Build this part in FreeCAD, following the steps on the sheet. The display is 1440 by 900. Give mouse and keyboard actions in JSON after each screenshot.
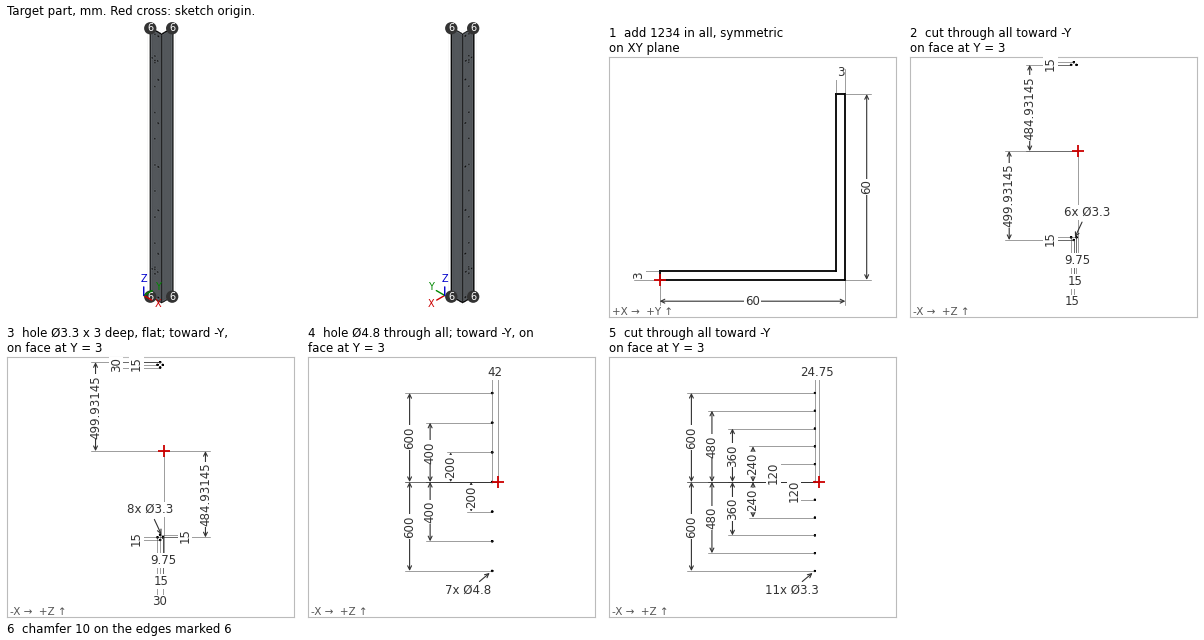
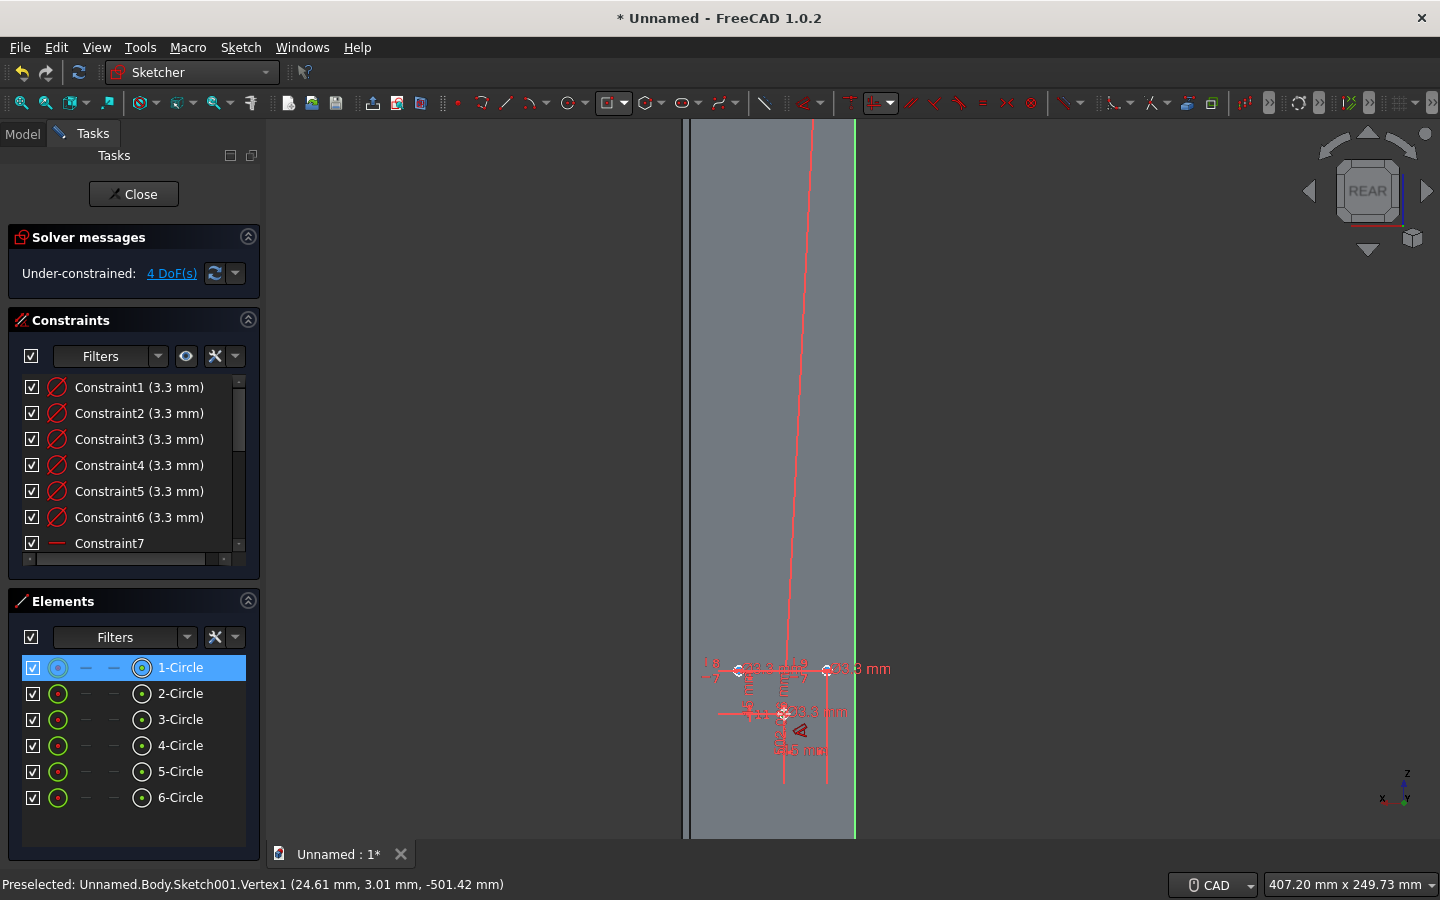
{"action": "left_click", "coordinate": [739, 671]}
{"action": "left_click", "coordinate": [761, 637]}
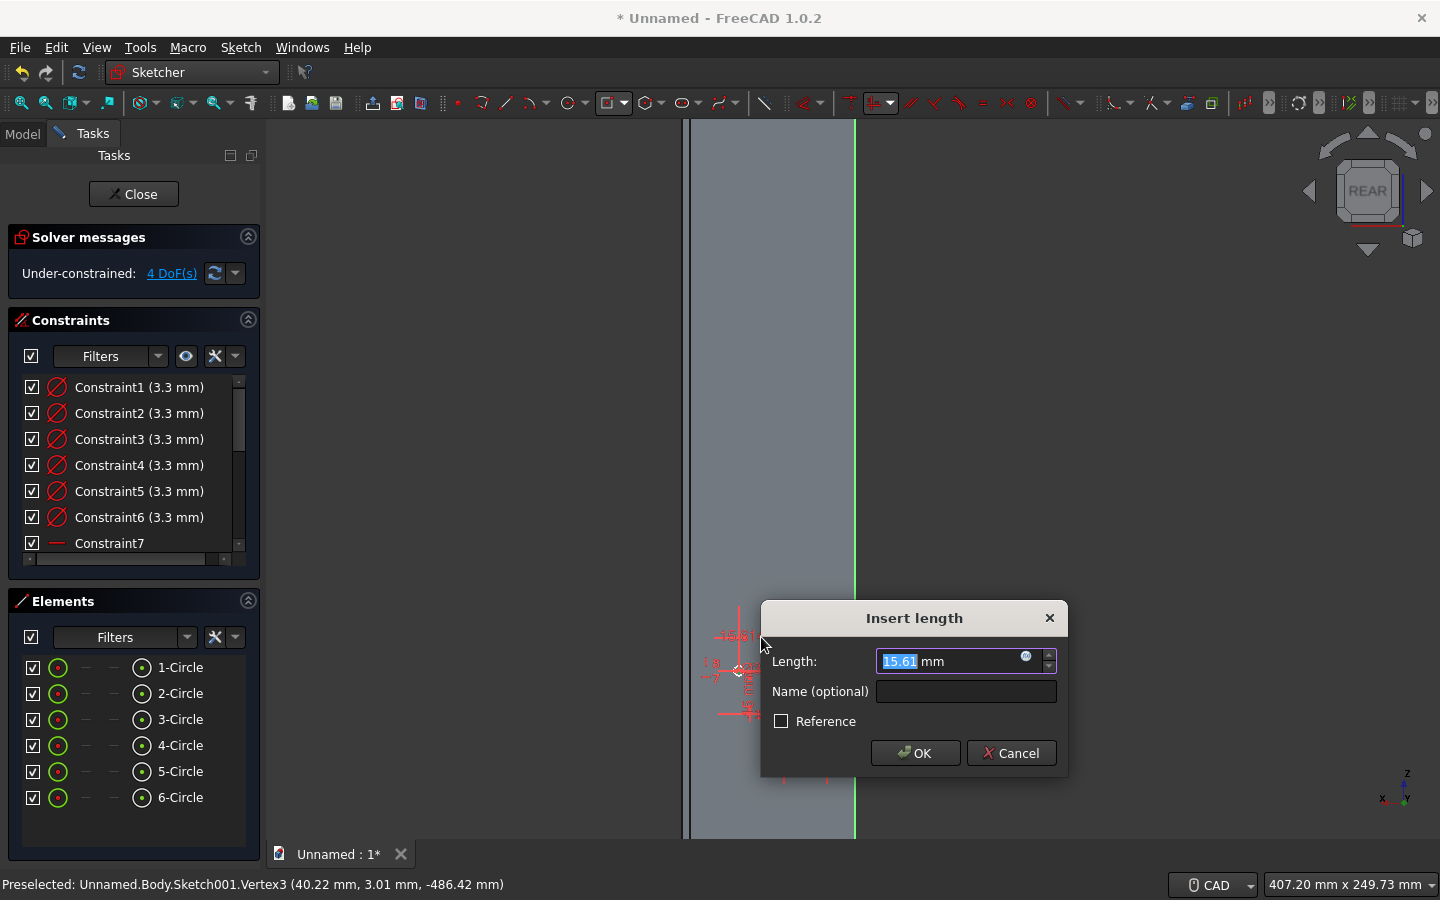
{"action": "type", "text": "15"}
{"action": "key", "text": "Return"}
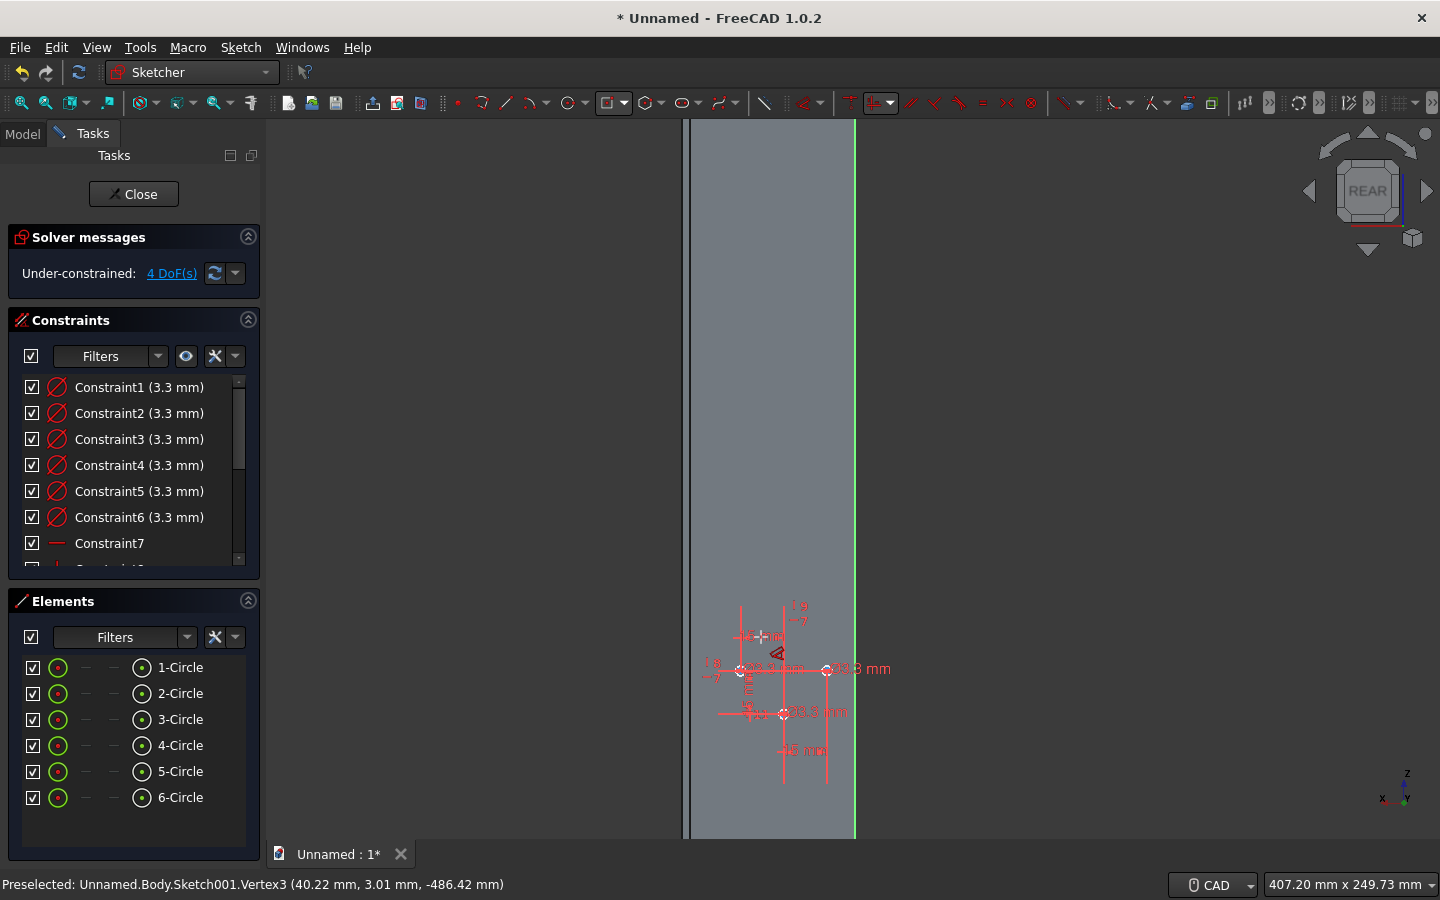
{"action": "scroll", "coordinate": [782, 719], "scroll_direction": "down", "scroll_amount": 9}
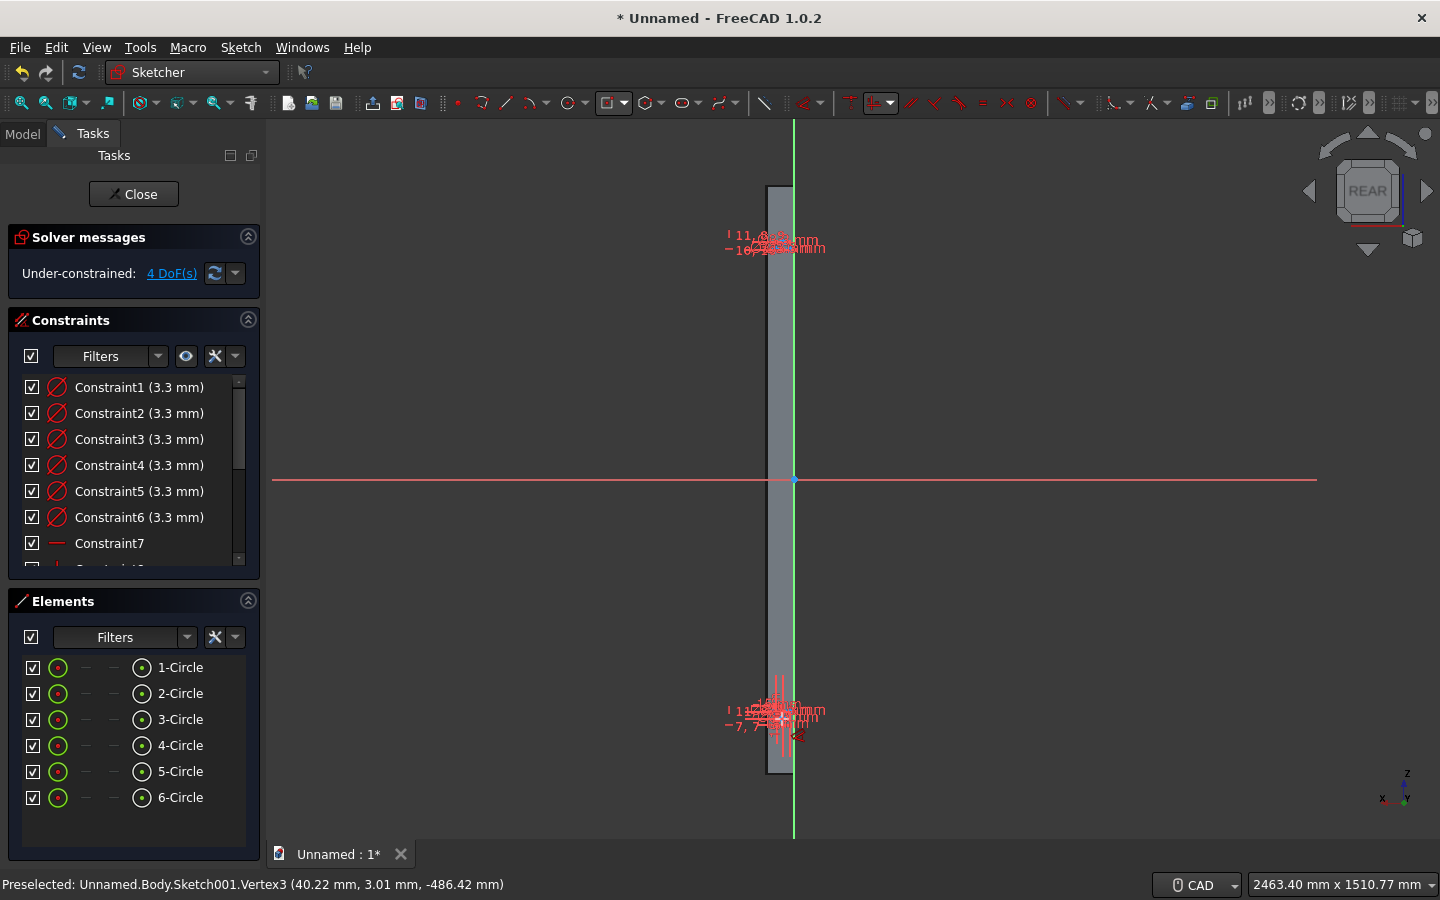
{"action": "scroll", "coordinate": [776, 250], "scroll_direction": "up", "scroll_amount": 9}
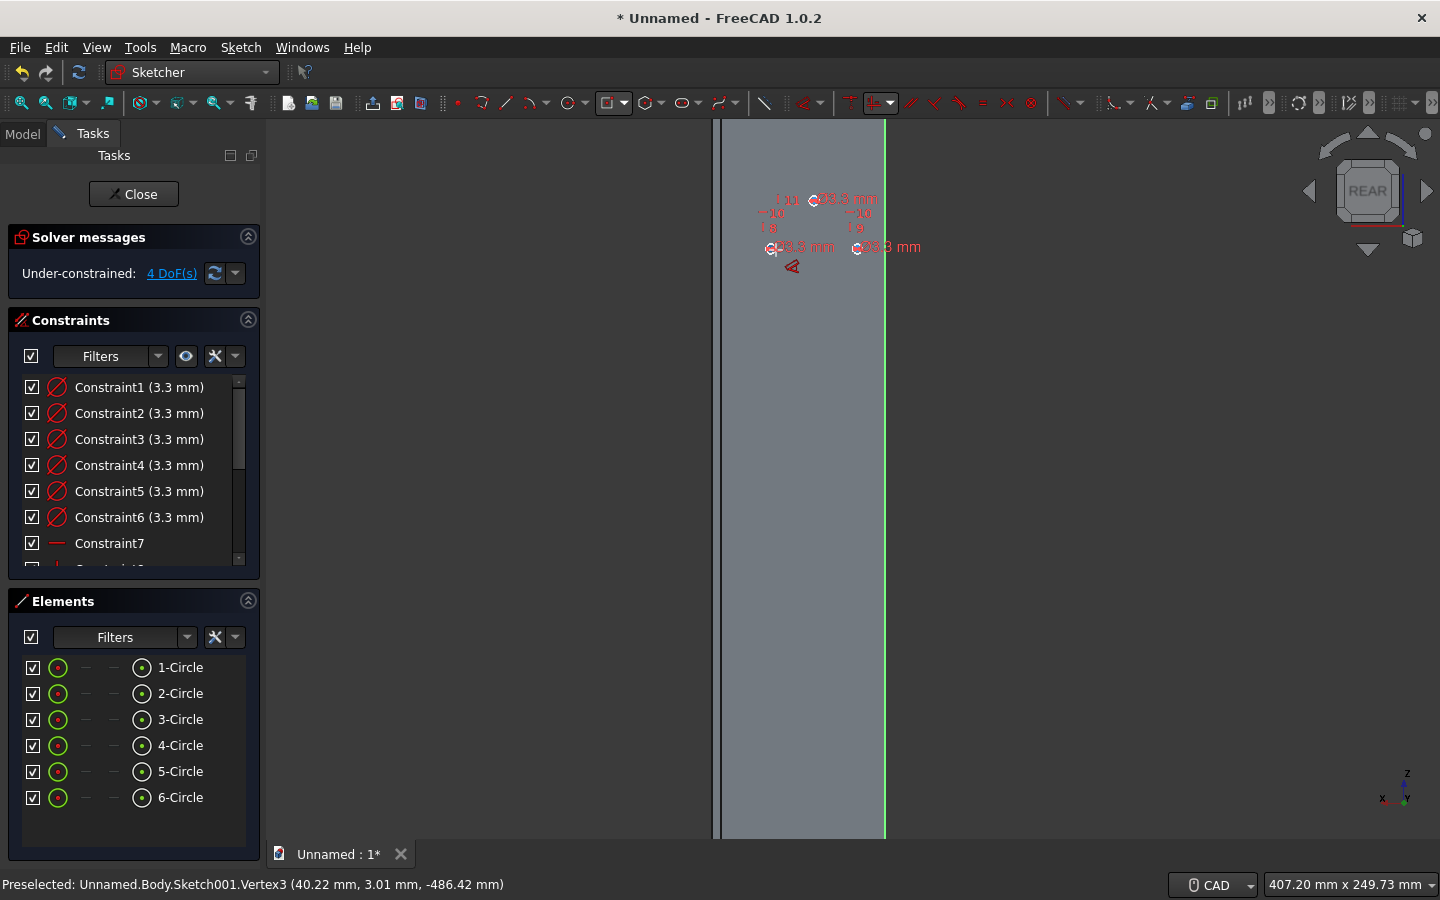
{"action": "left_click", "coordinate": [771, 249]}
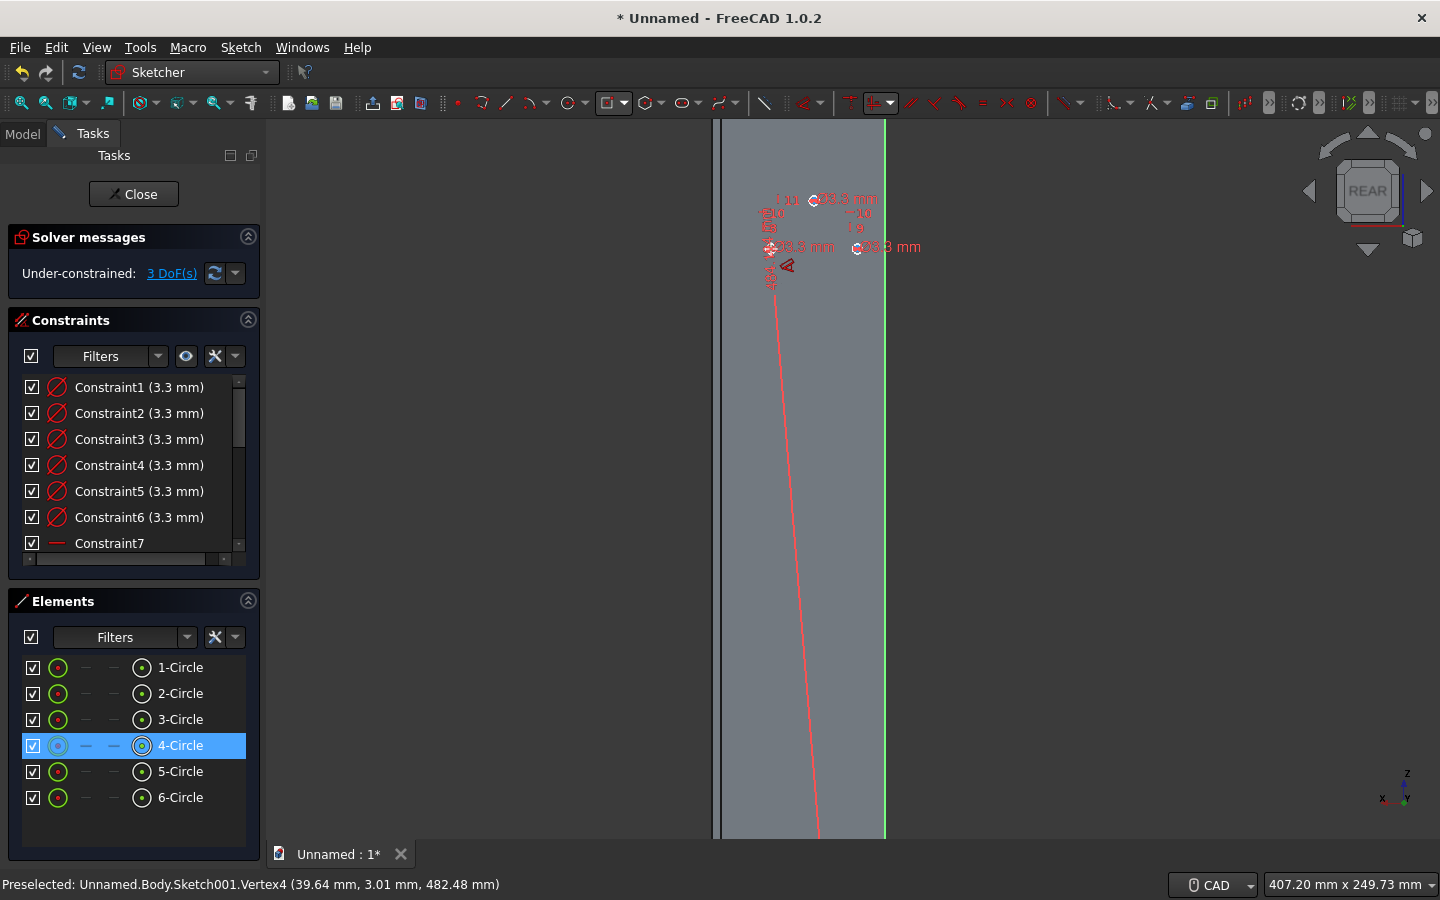
{"action": "left_click", "coordinate": [814, 201]}
{"action": "left_click", "coordinate": [737, 225]}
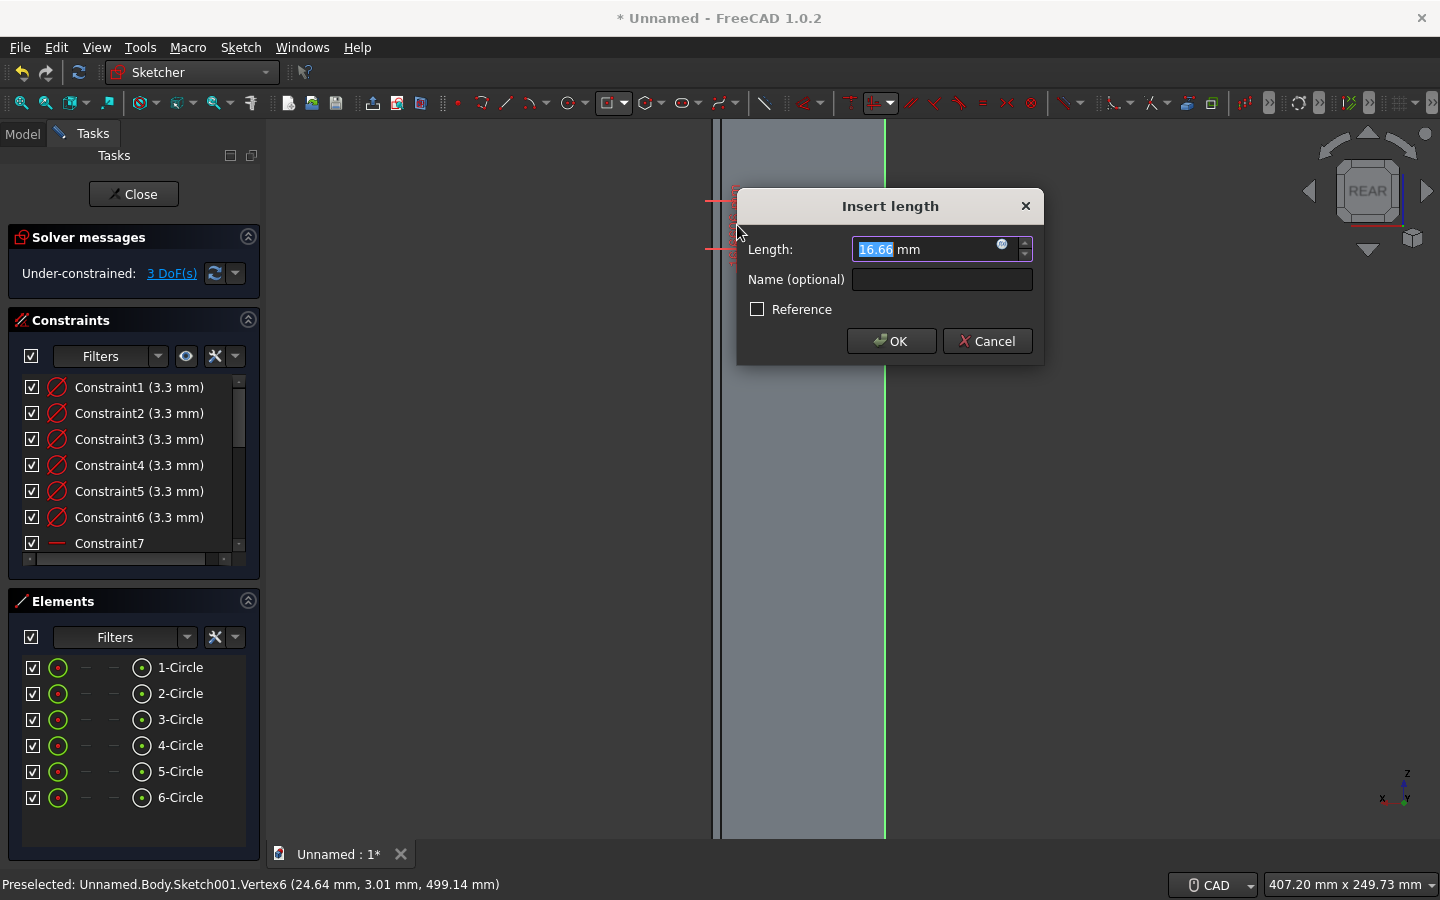
{"action": "type", "text": "15"}
{"action": "key", "text": "Return"}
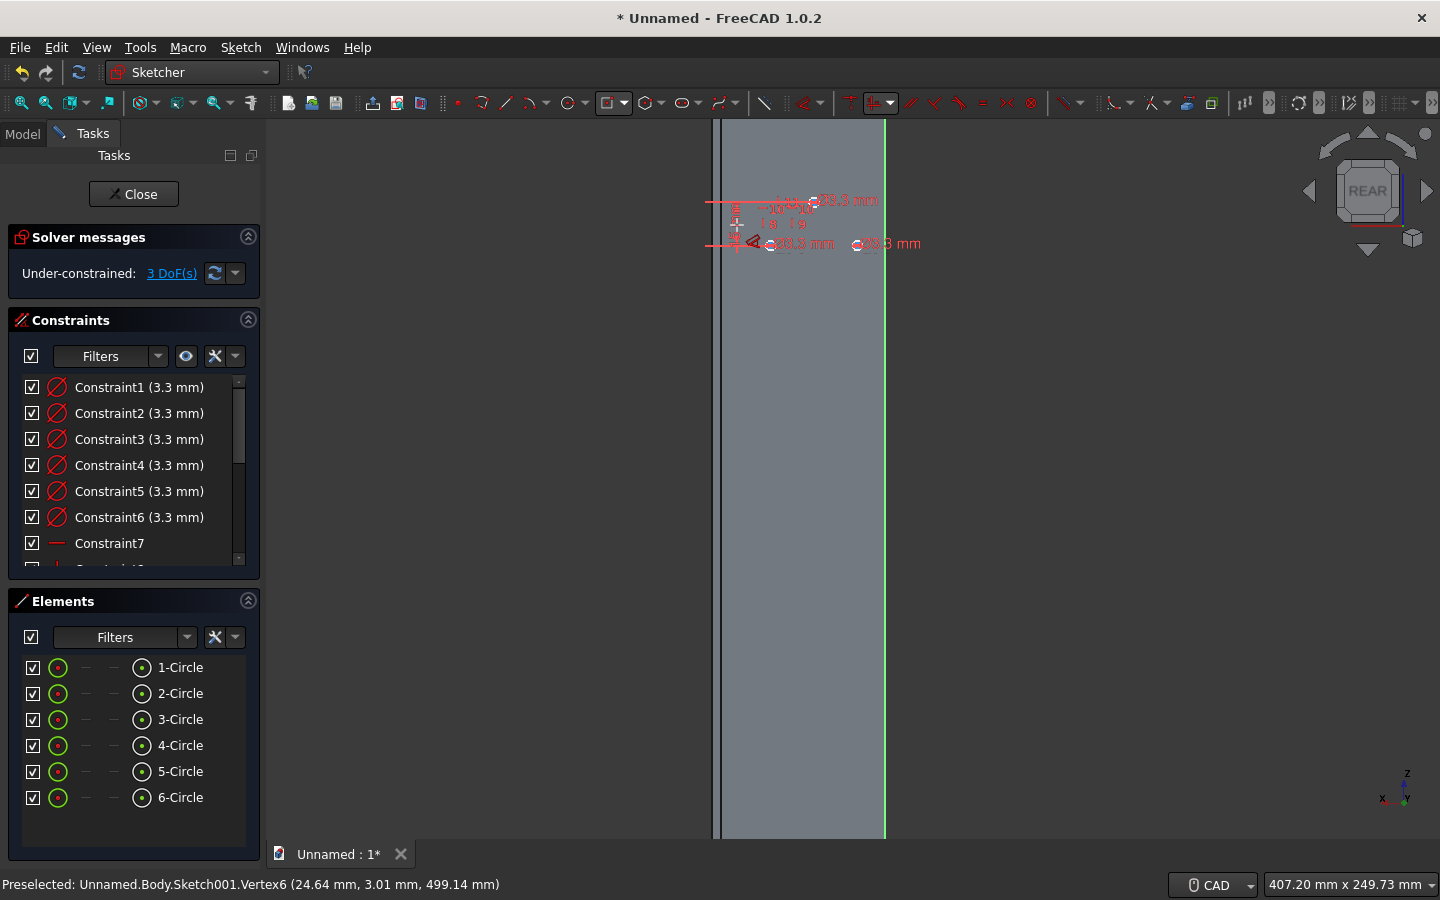
{"action": "scroll", "coordinate": [776, 249], "scroll_direction": "down", "scroll_amount": 9}